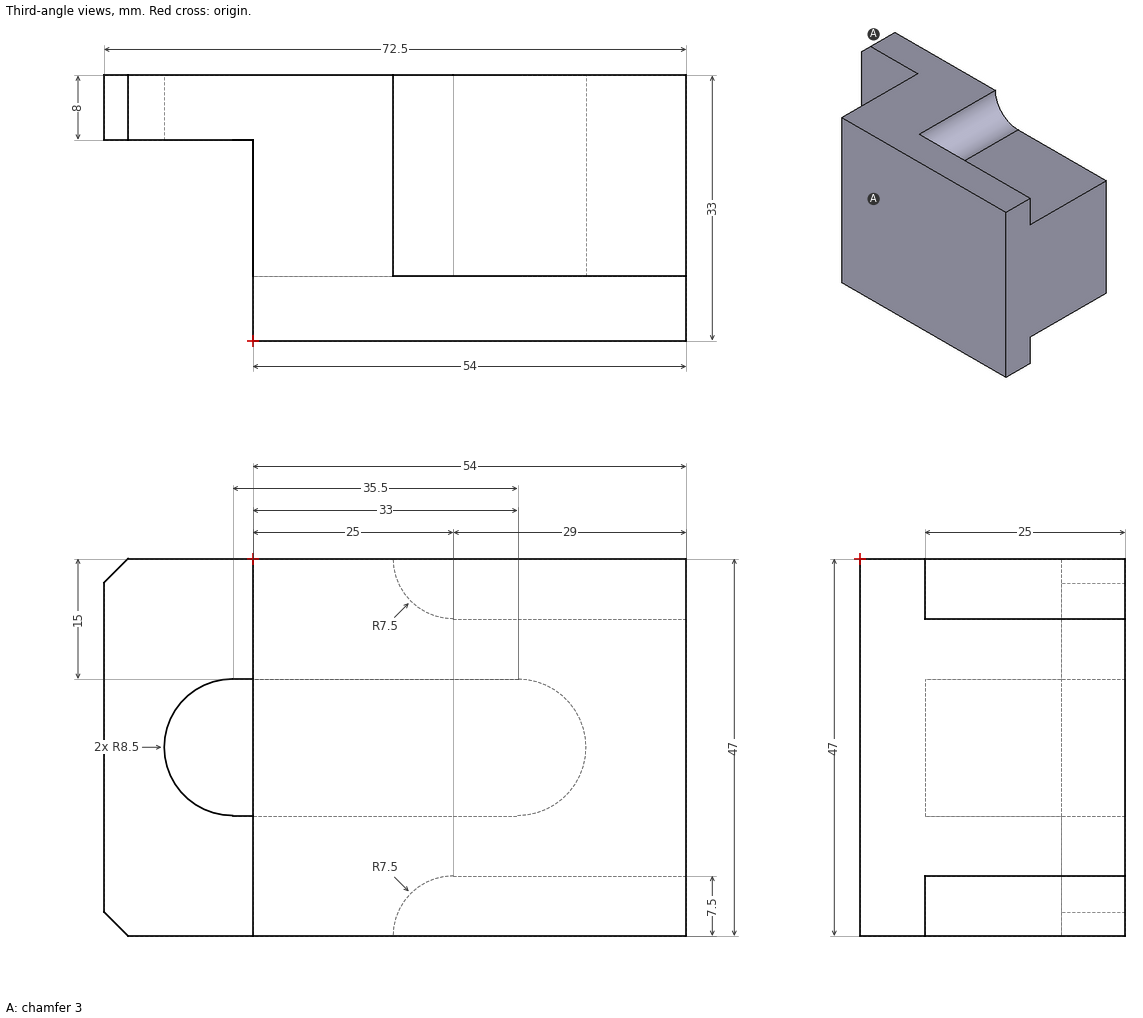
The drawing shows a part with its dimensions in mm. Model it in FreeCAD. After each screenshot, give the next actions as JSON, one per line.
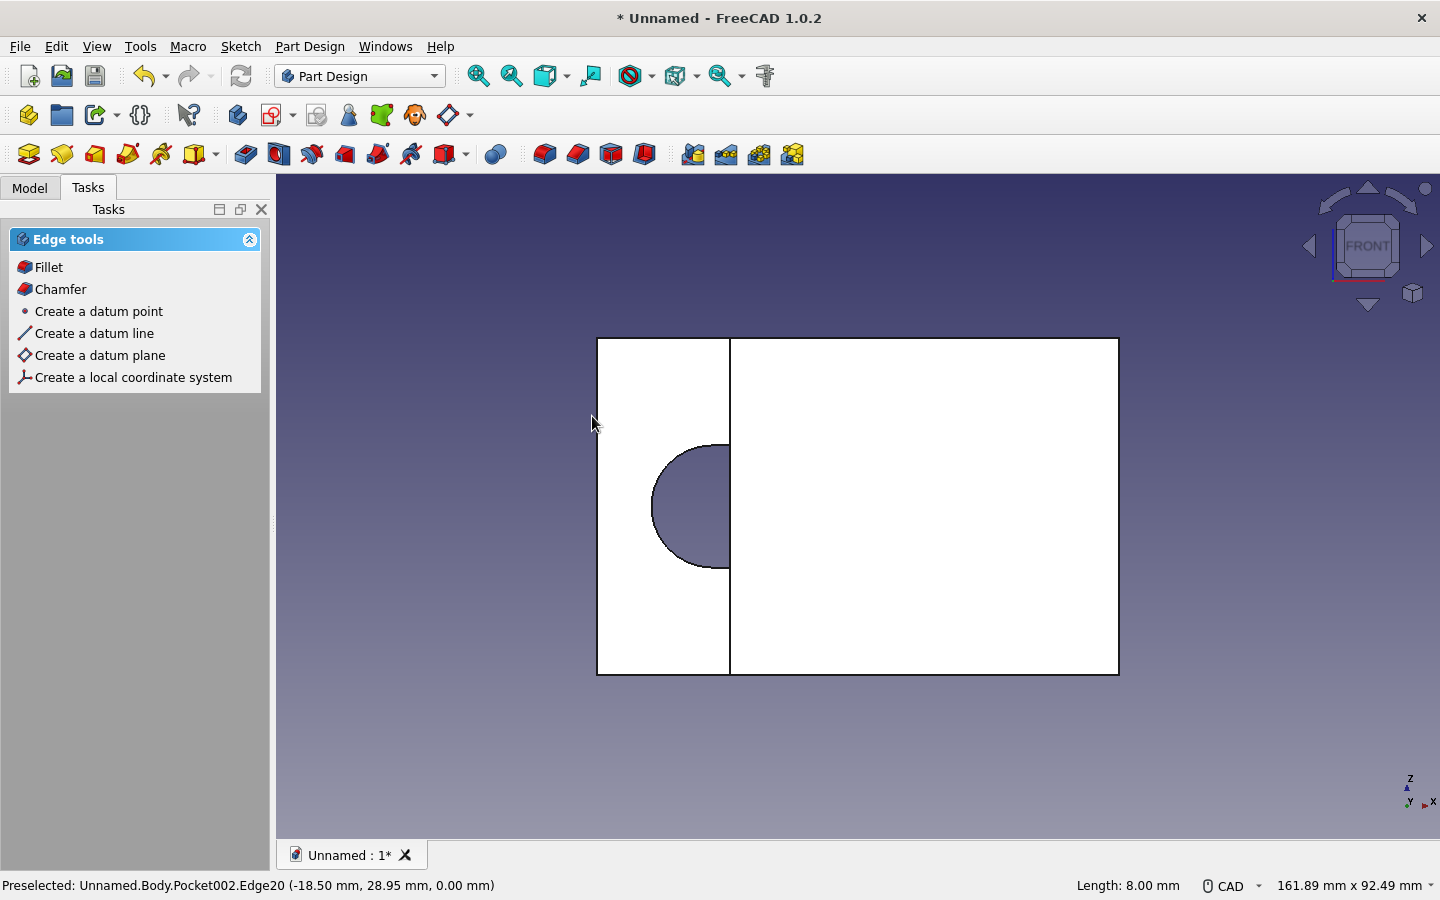
{"action": "key", "text": "3"}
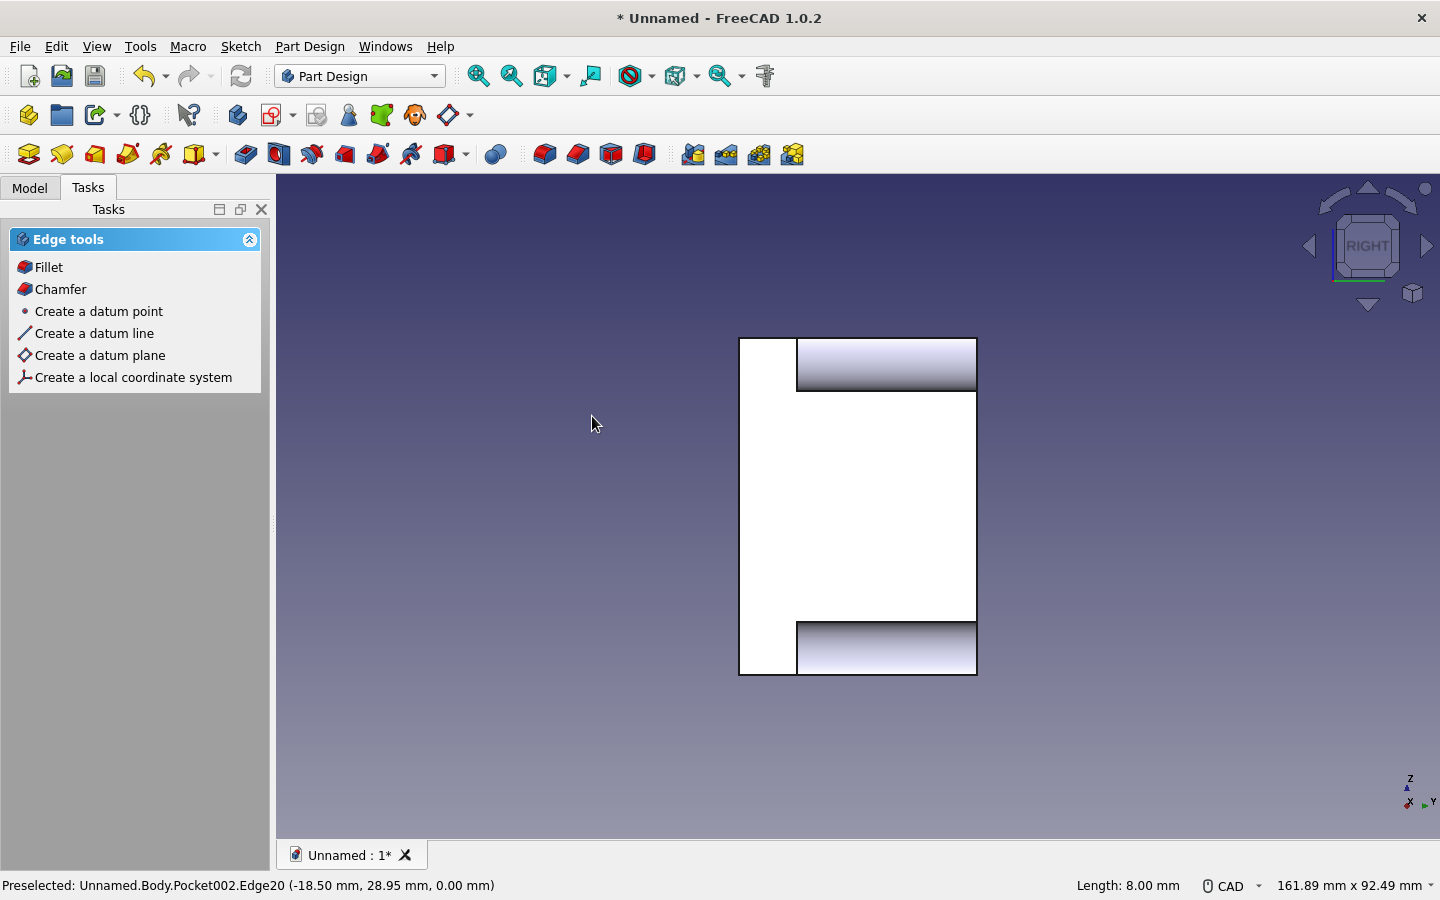
{"action": "key", "text": "5"}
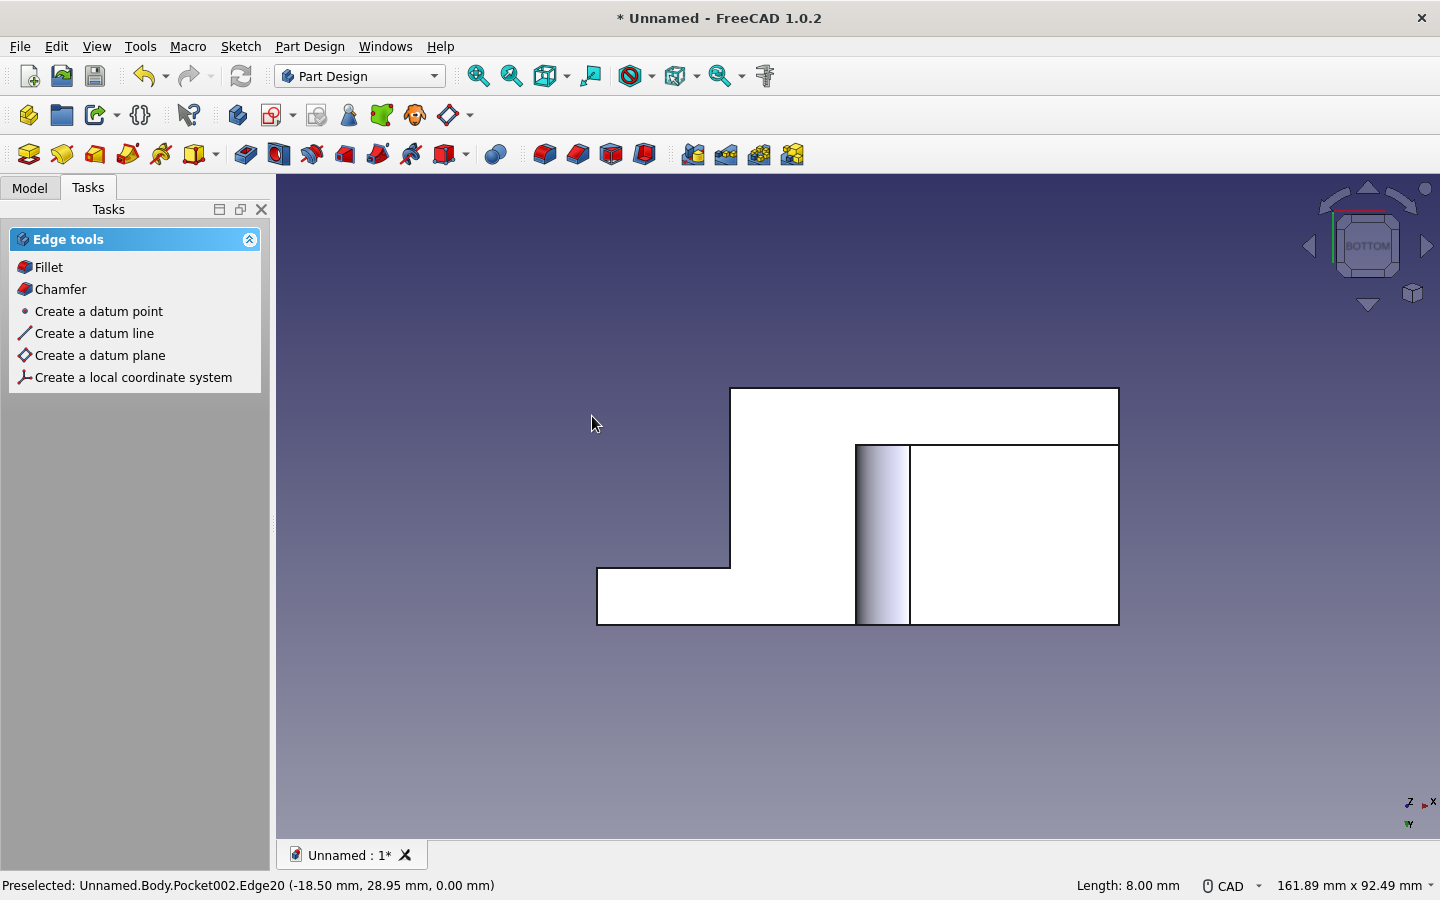
{"action": "left_click", "coordinate": [479, 76]}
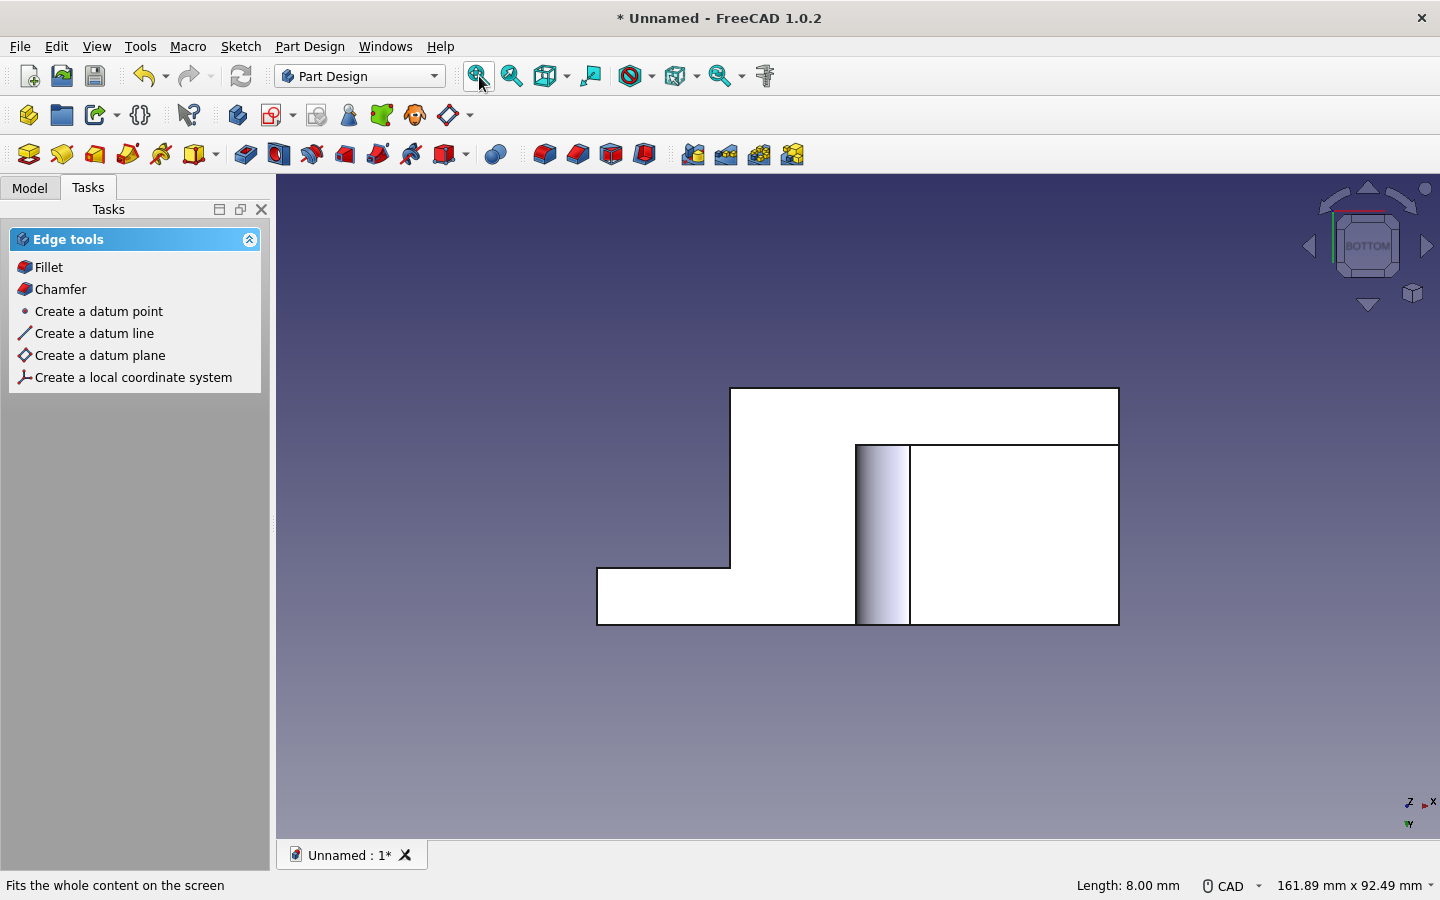
{"action": "left_click", "coordinate": [597, 595], "text": "ctrl"}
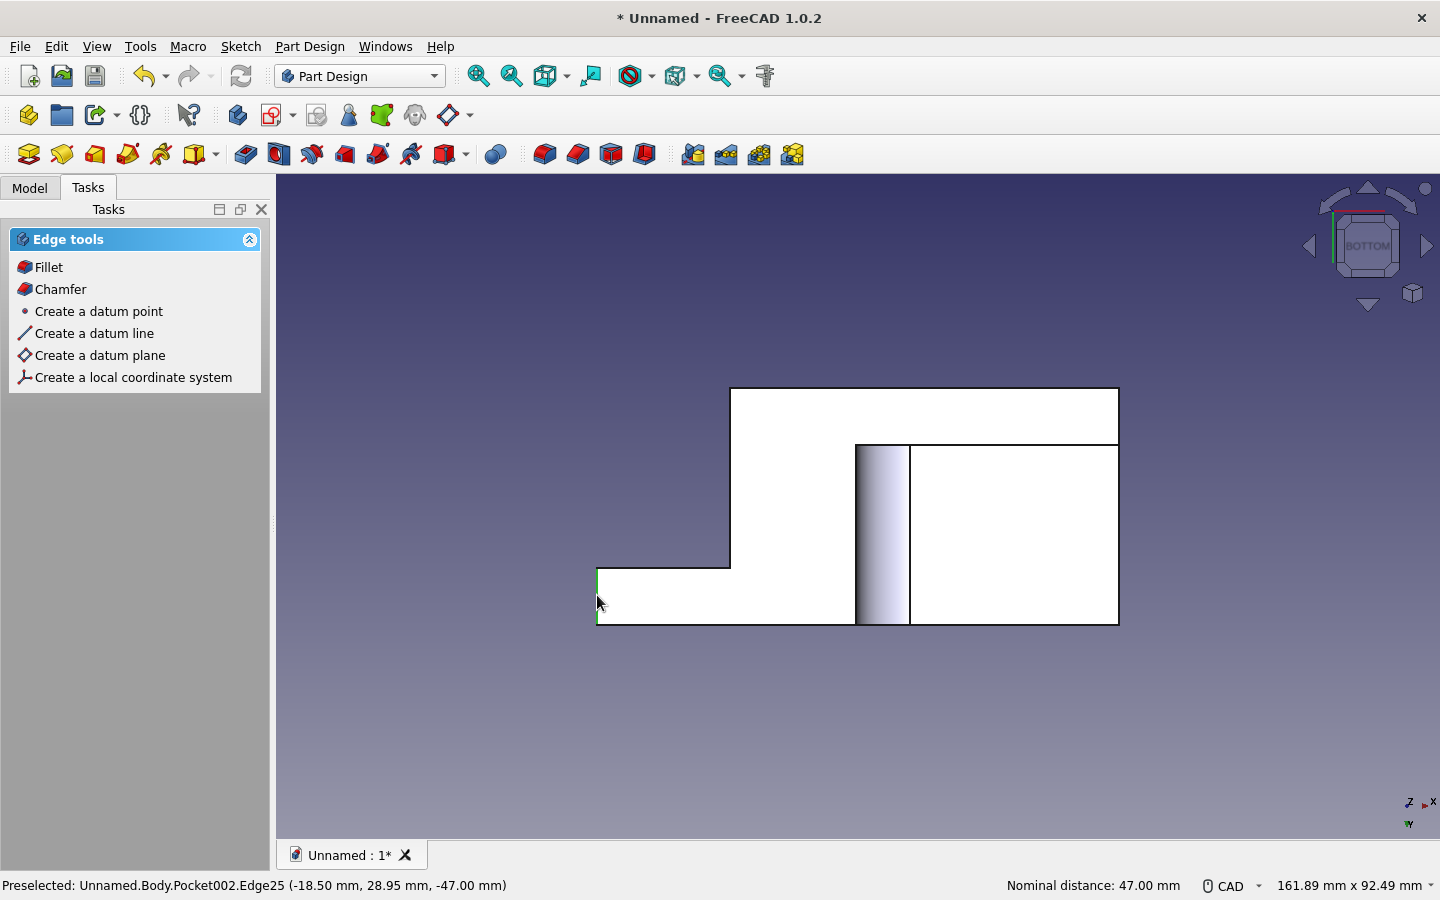
{"action": "left_click", "coordinate": [578, 154]}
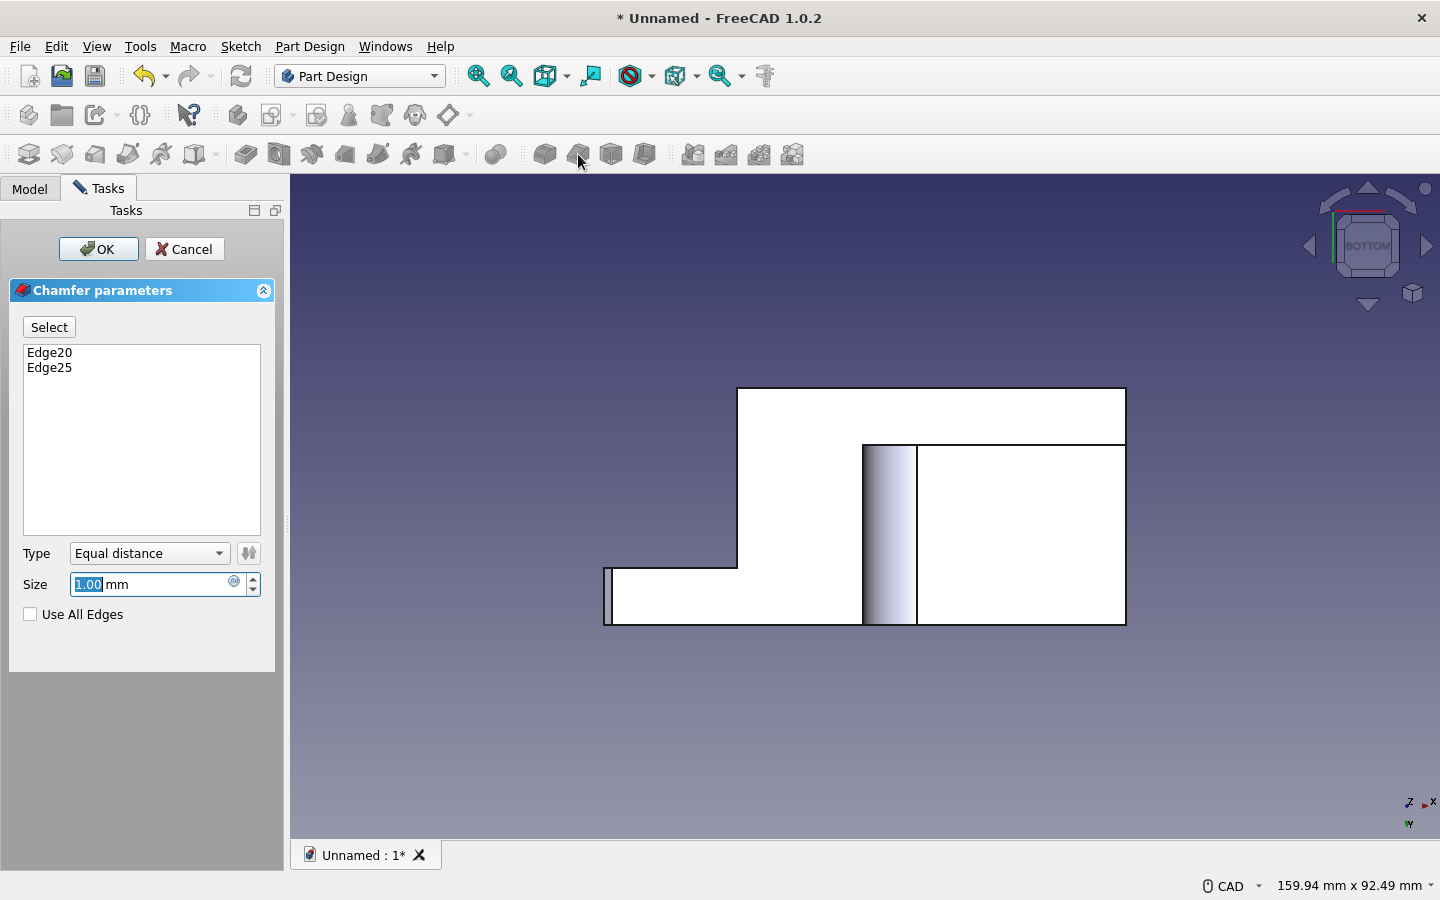
{"action": "type", "text": "3"}
{"action": "key", "text": "Tab"}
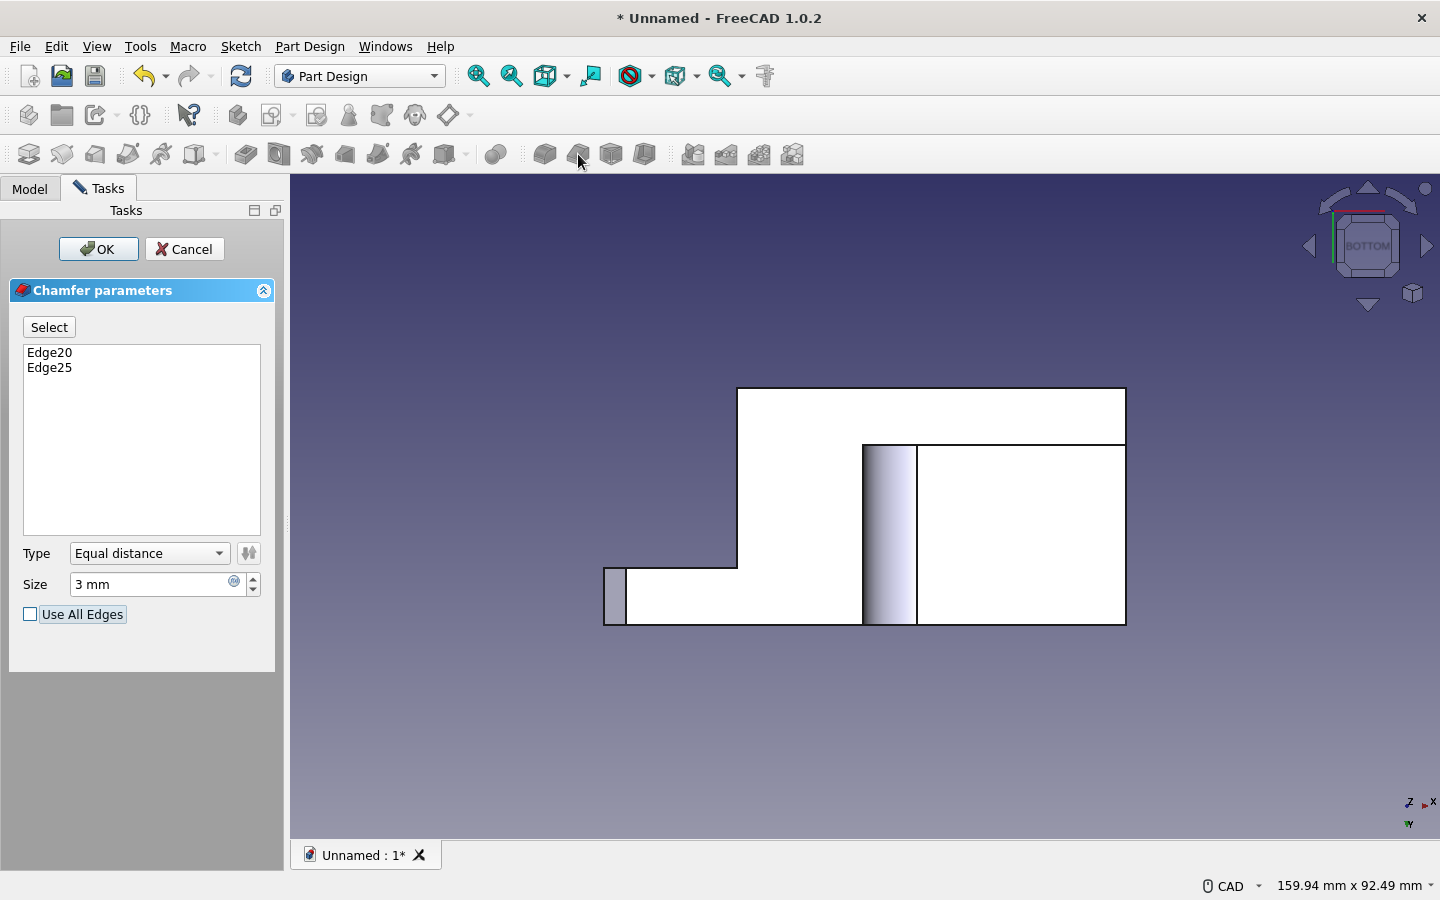
{"action": "left_click", "coordinate": [99, 249]}